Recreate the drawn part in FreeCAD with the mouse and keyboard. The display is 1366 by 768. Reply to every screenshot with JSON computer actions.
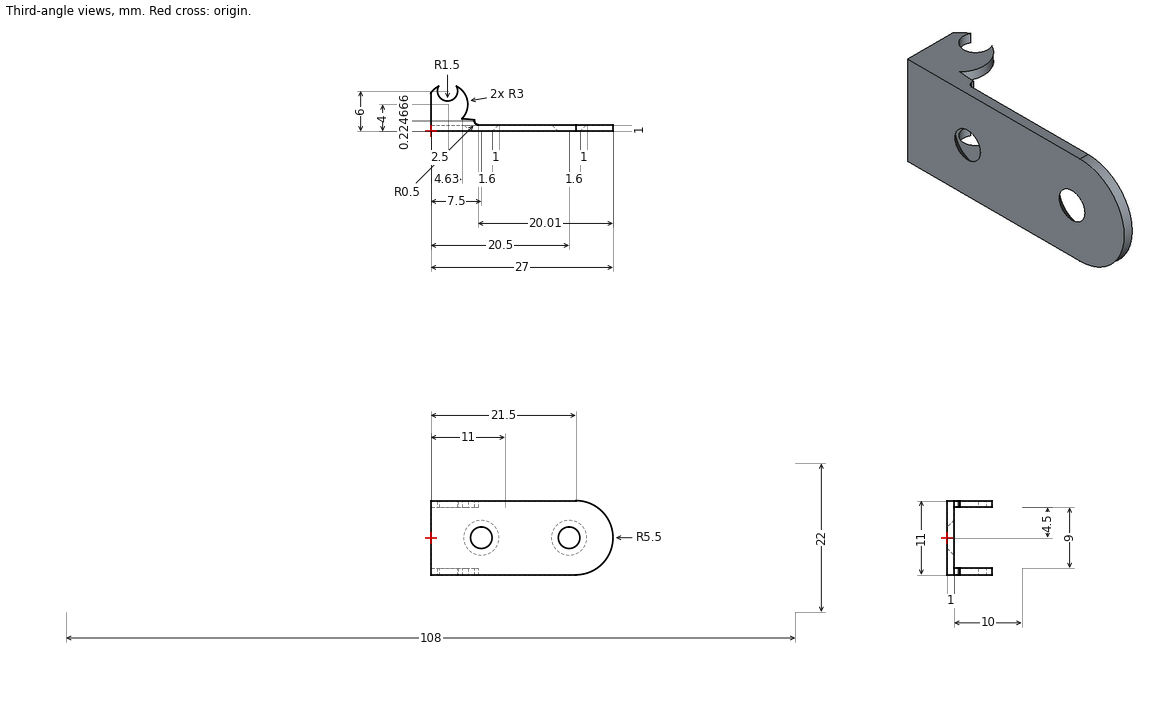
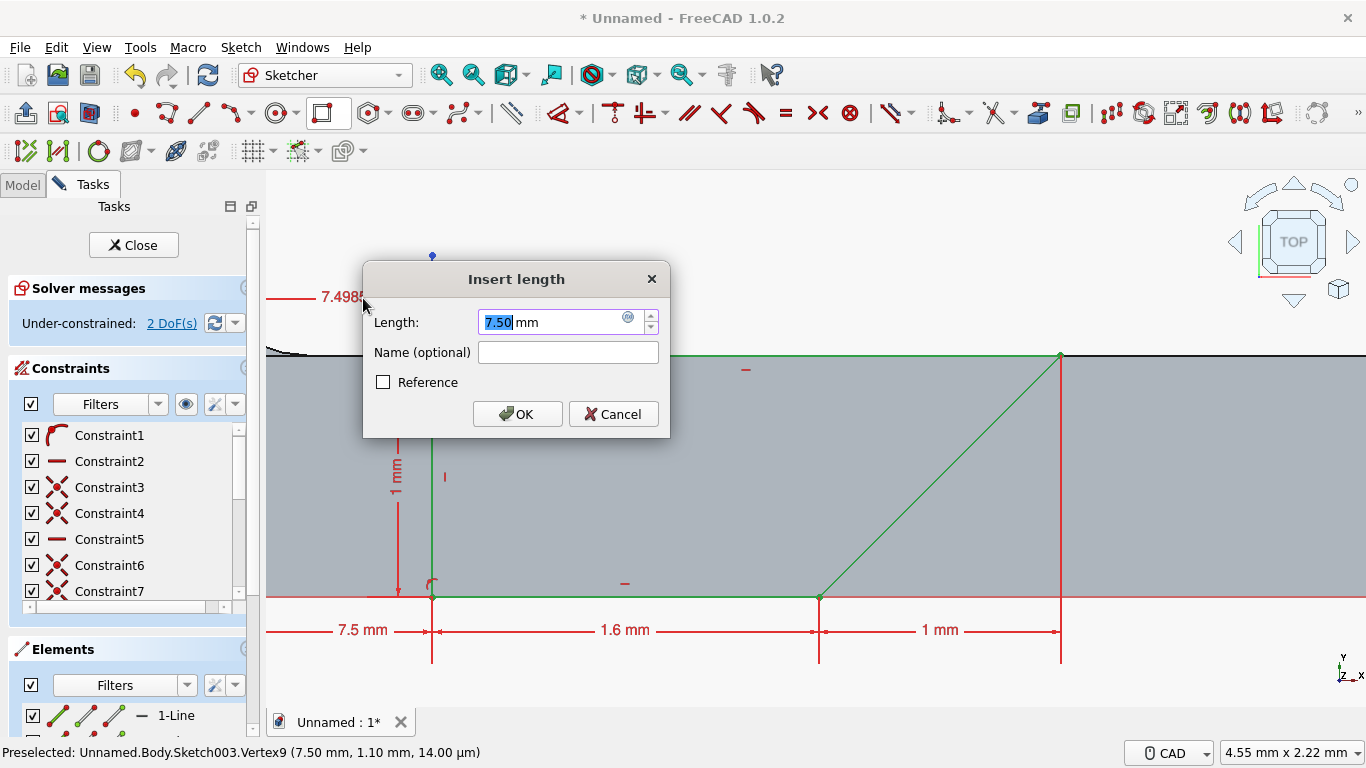
{"action": "type", "text": "7.5"}
{"action": "key", "text": "Return"}
{"action": "key", "text": "Escape"}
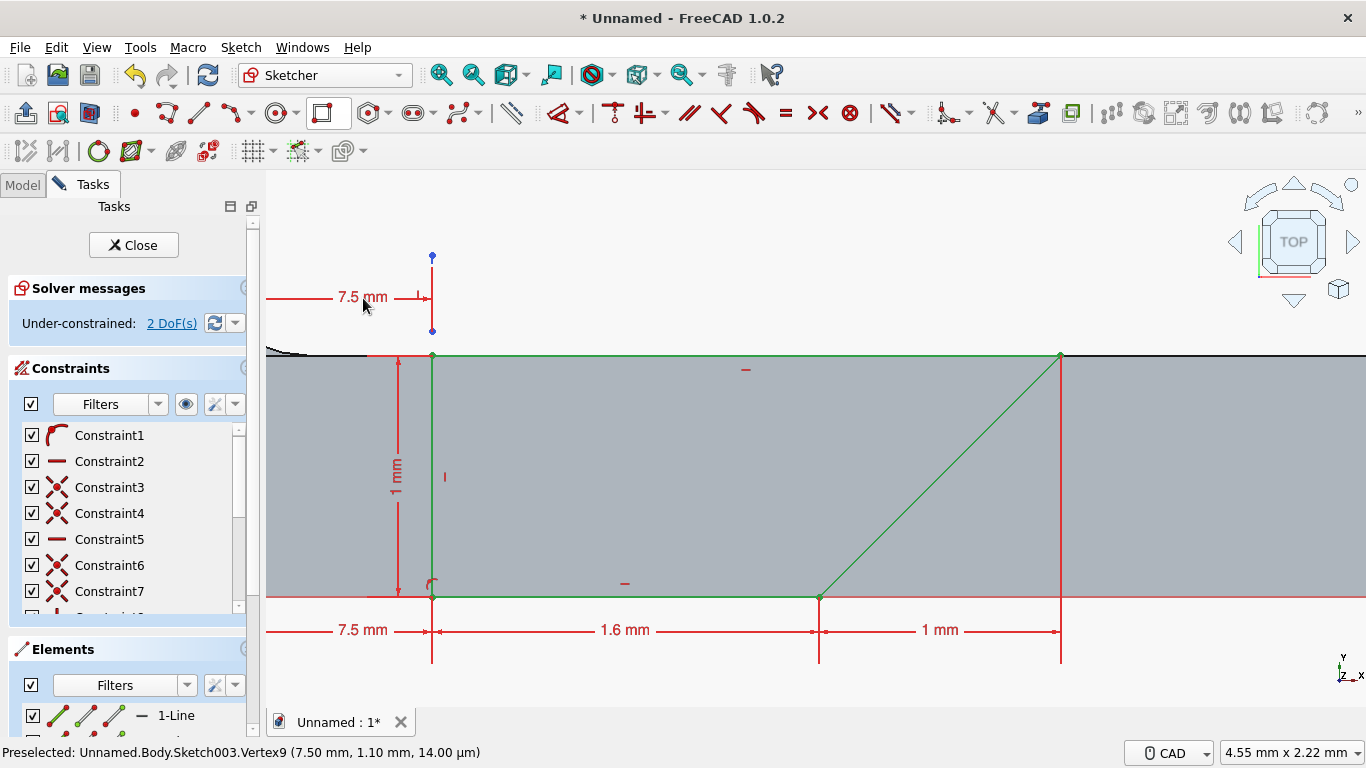
{"action": "left_click", "coordinate": [134, 245]}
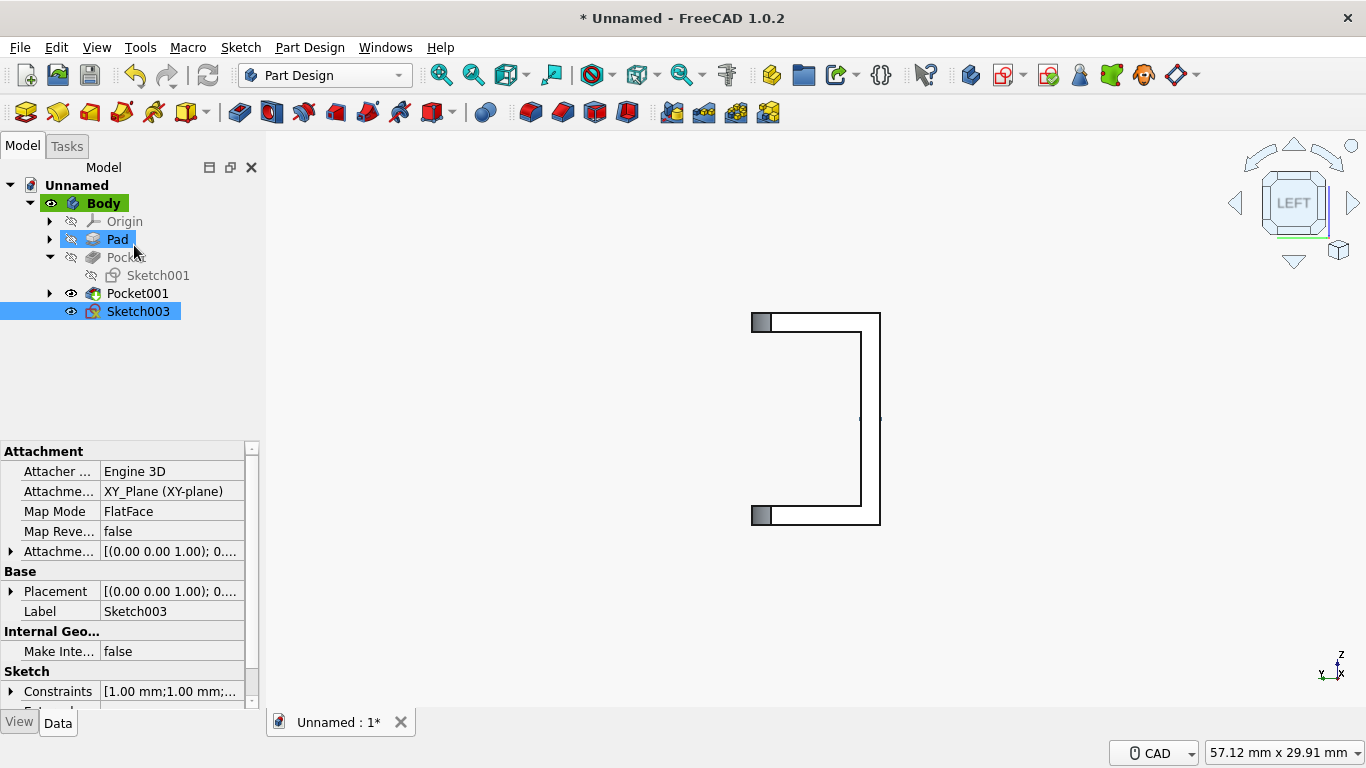
{"action": "left_click", "coordinate": [304, 112]}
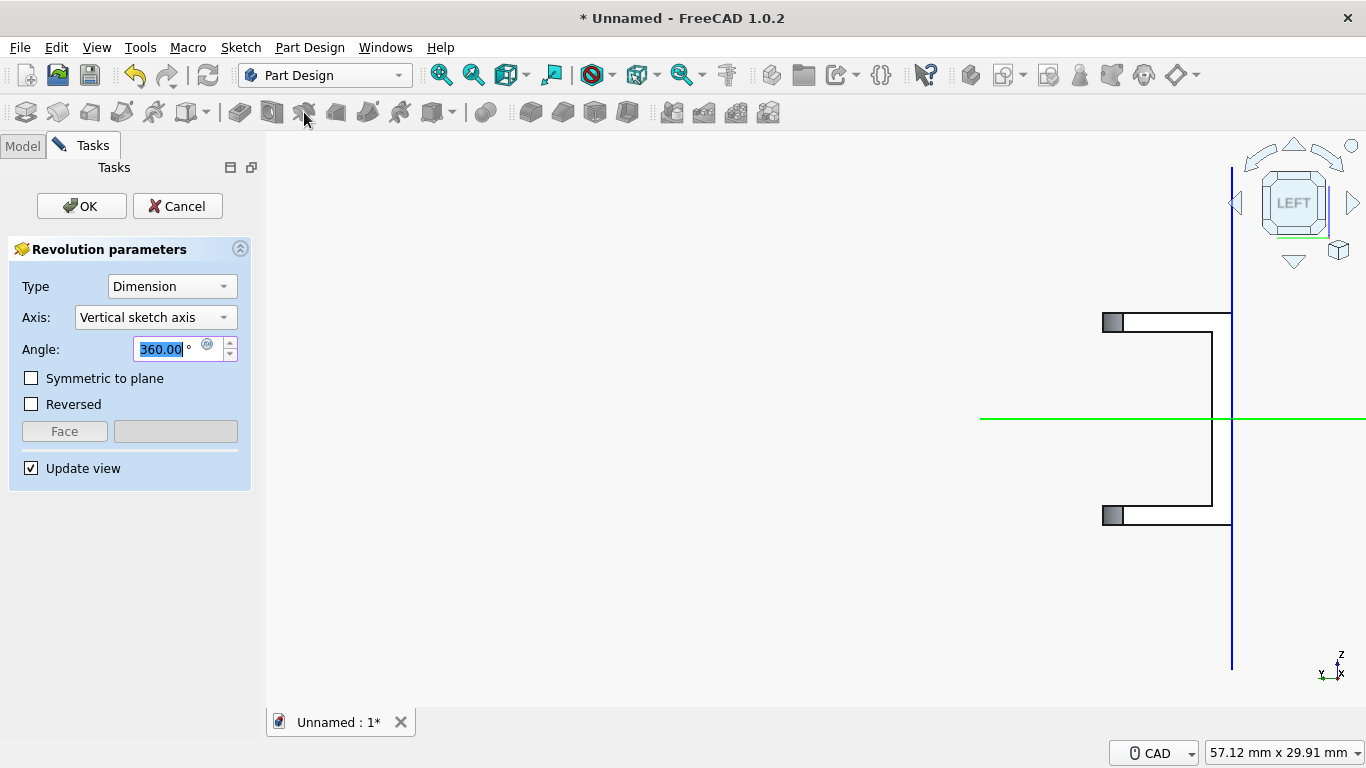
{"action": "left_click", "coordinate": [156, 318]}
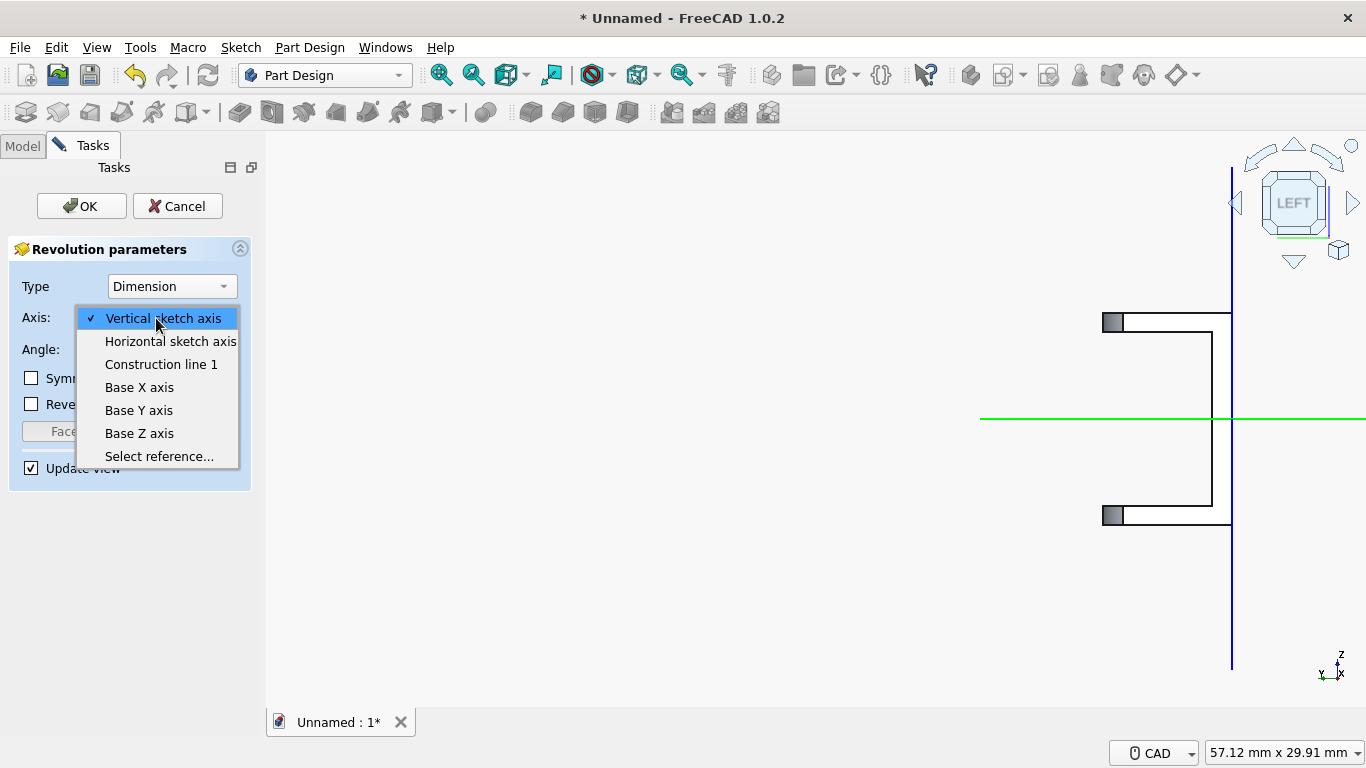
{"action": "left_click", "coordinate": [156, 364]}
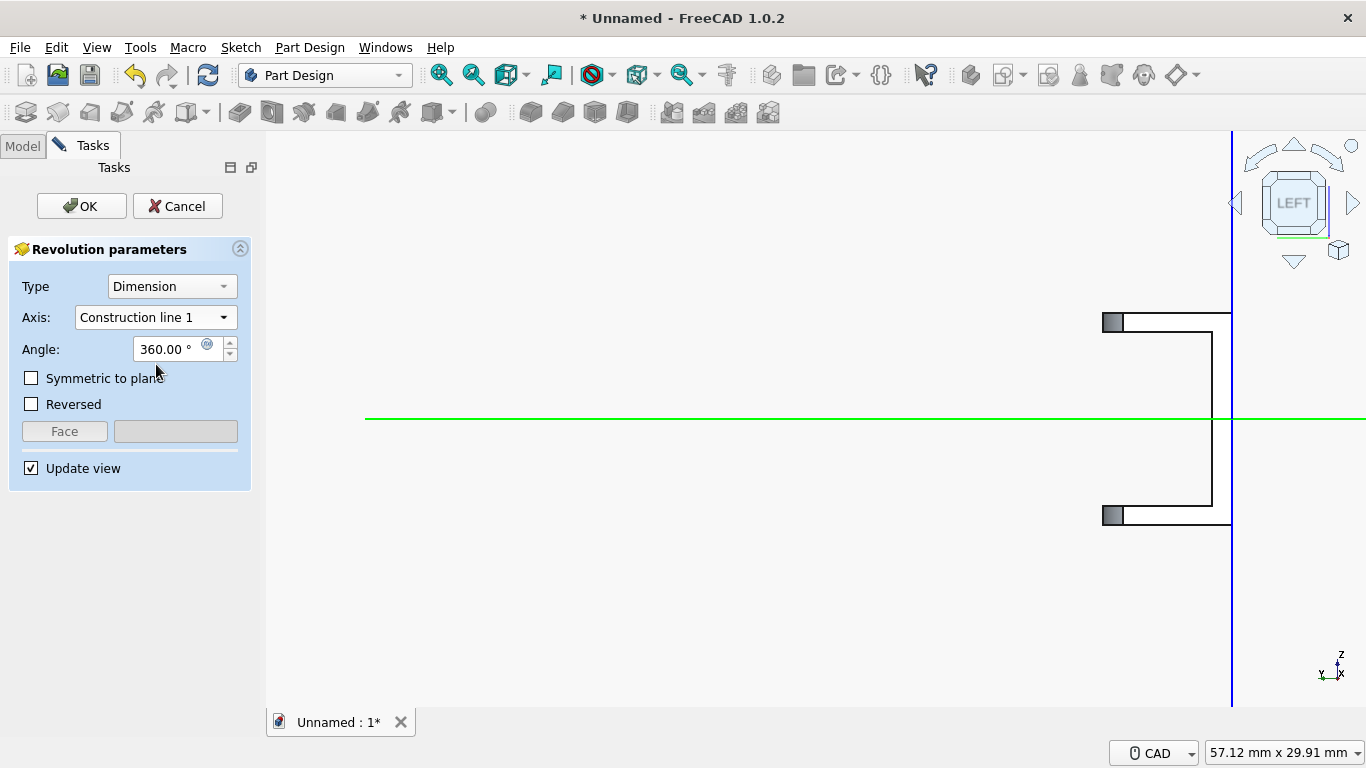
{"action": "left_click", "coordinate": [82, 206]}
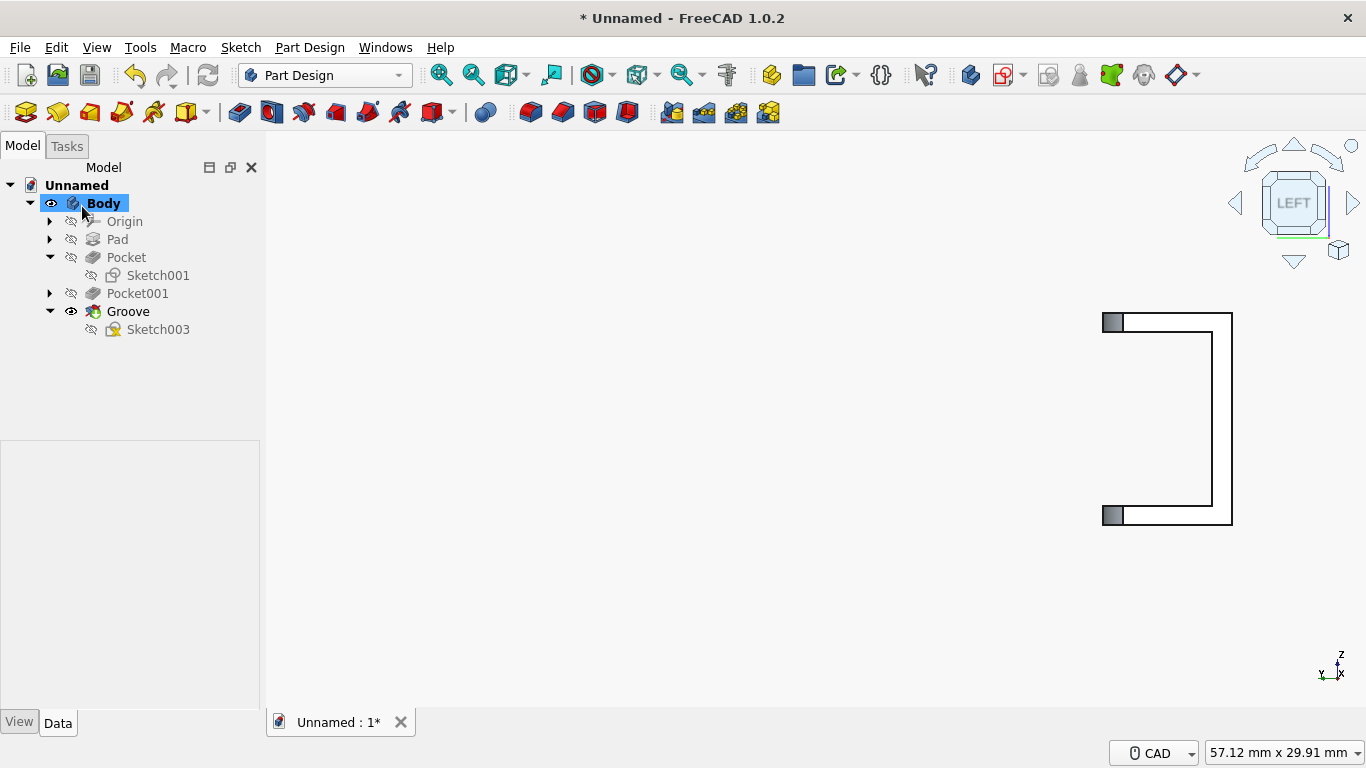
{"action": "left_click", "coordinate": [442, 76]}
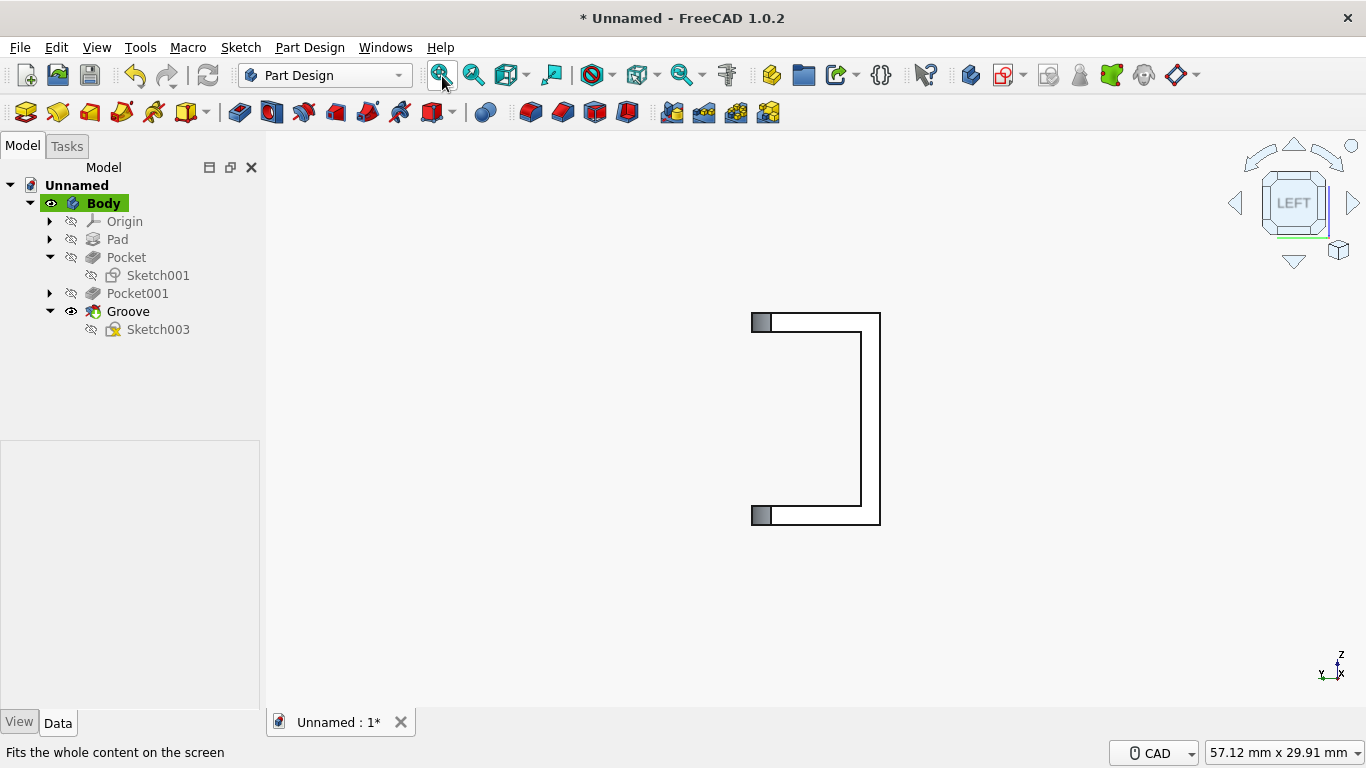
{"action": "left_click", "coordinate": [1004, 76]}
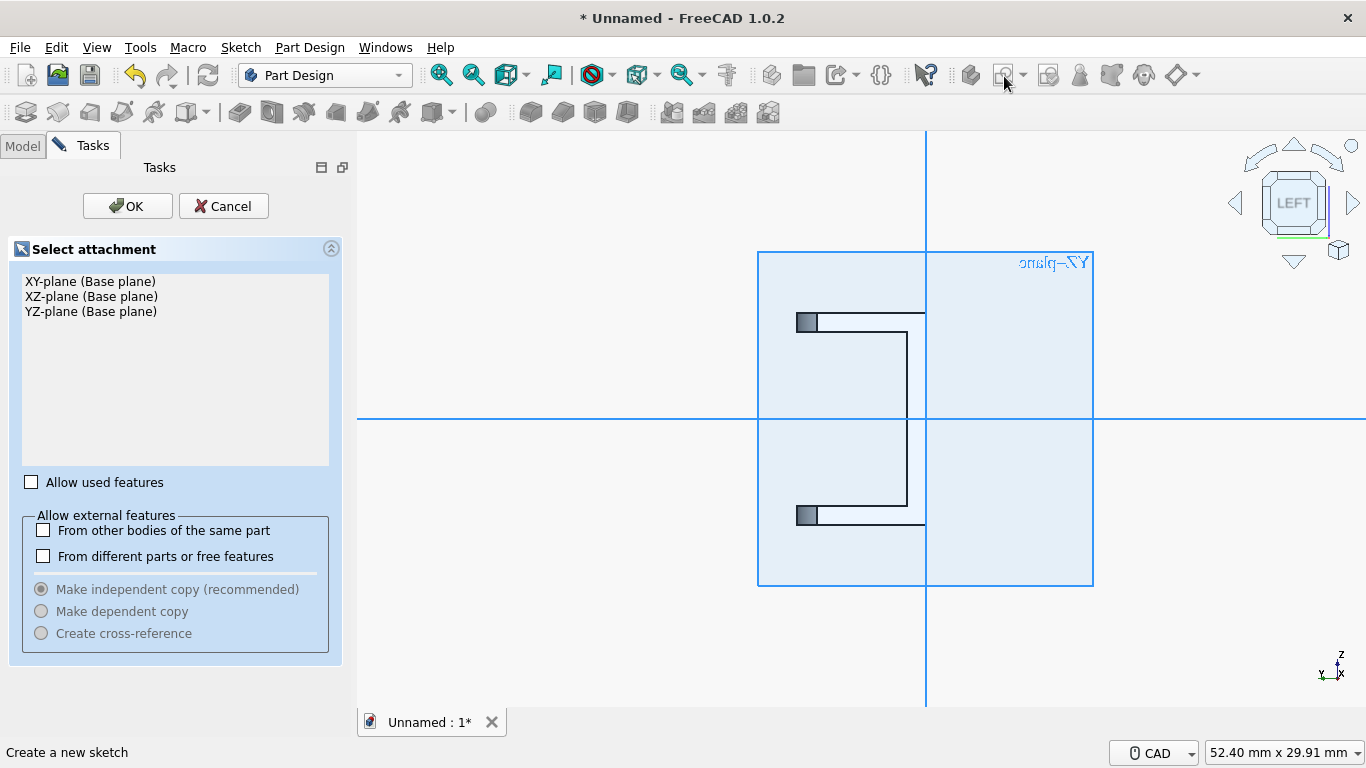
{"action": "left_click", "coordinate": [82, 282]}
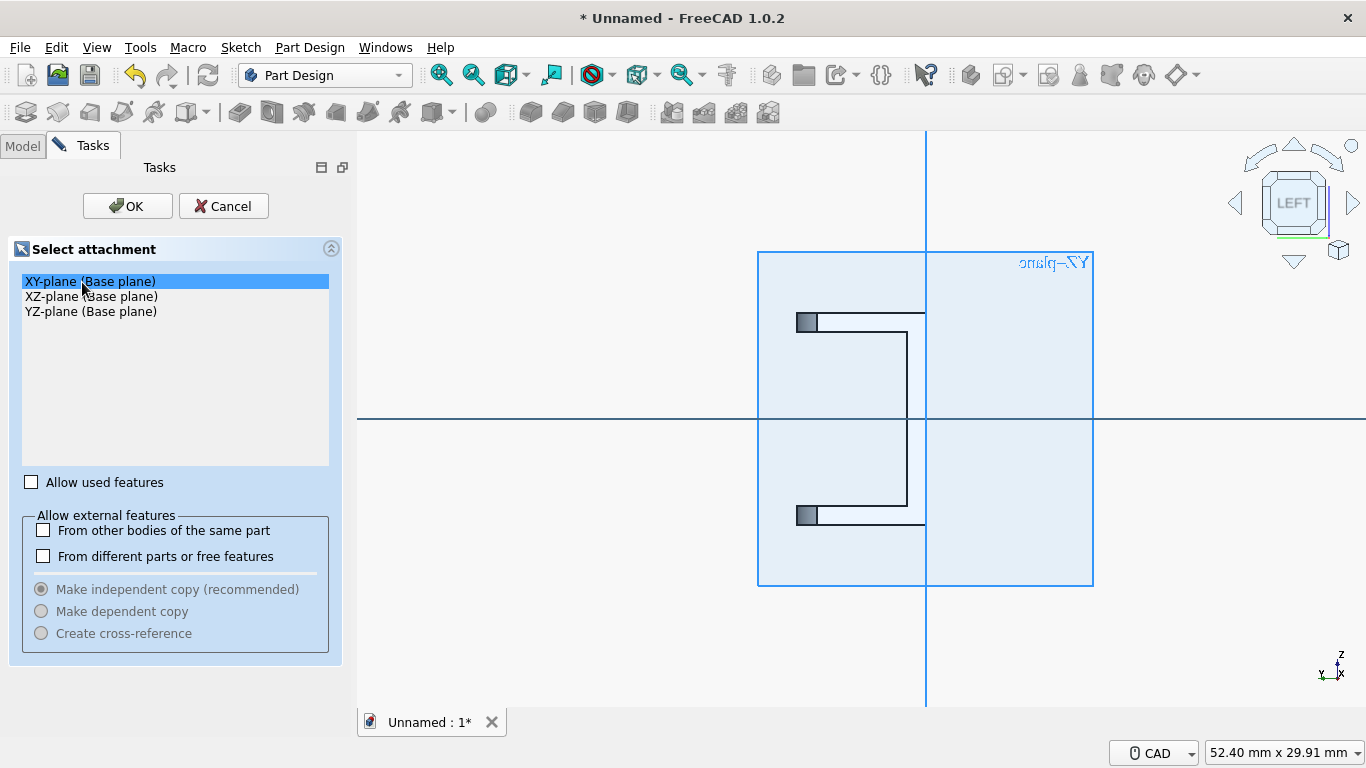
{"action": "left_click", "coordinate": [128, 206]}